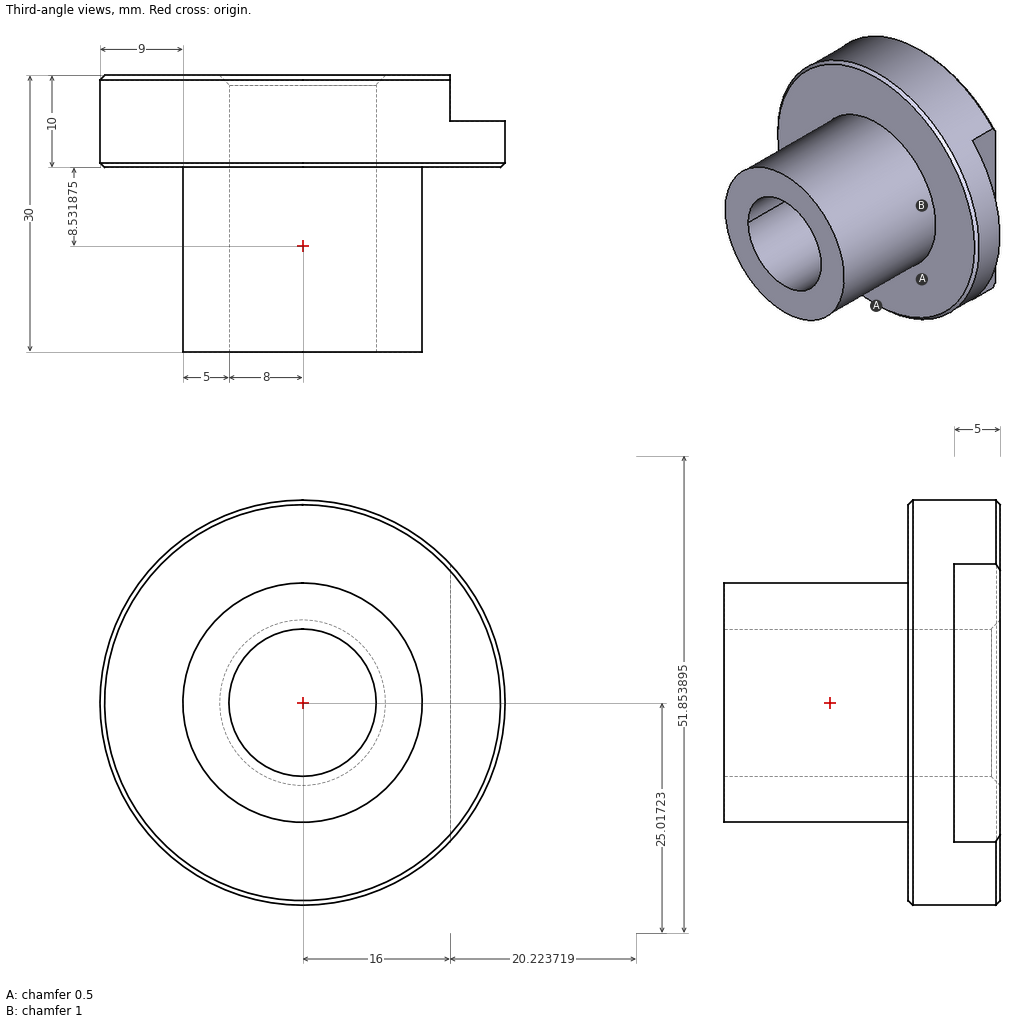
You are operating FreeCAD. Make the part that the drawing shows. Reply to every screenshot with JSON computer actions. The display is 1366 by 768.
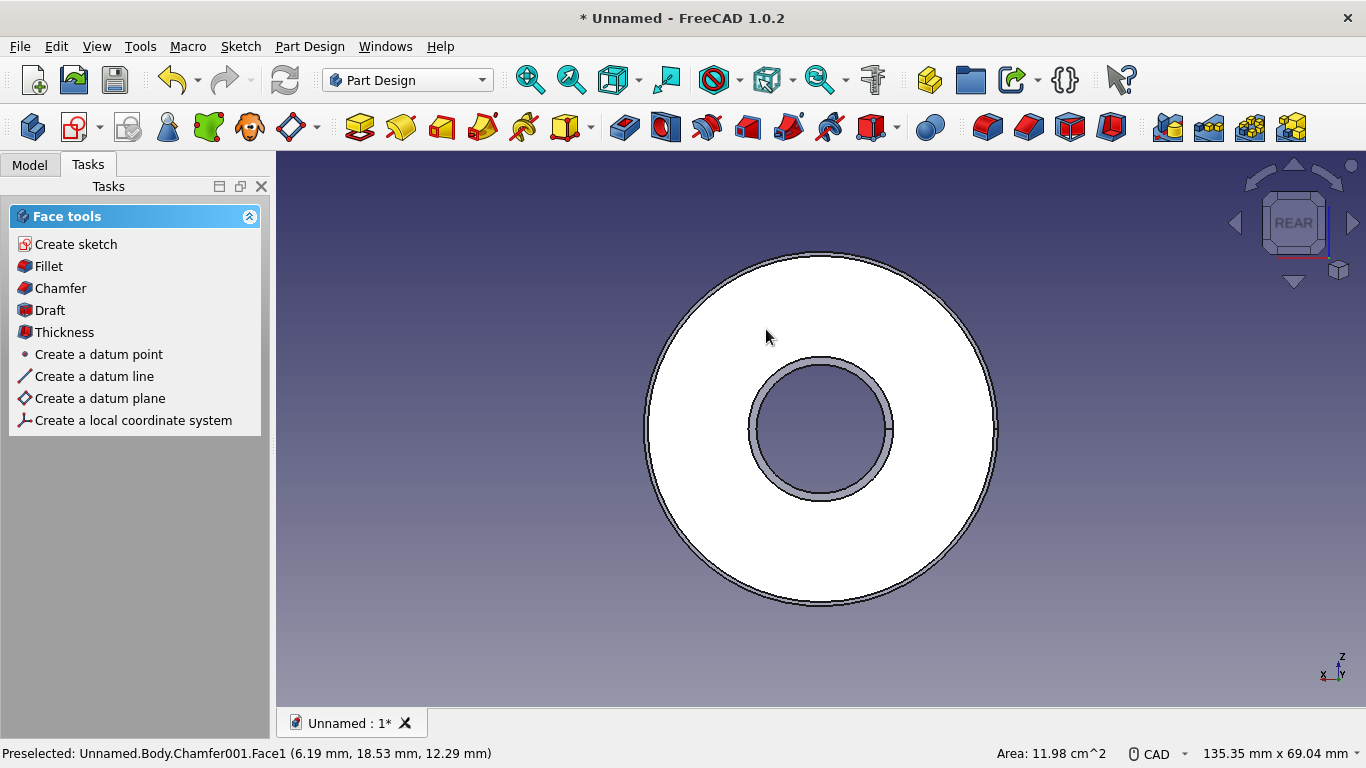
{"action": "left_click", "coordinate": [74, 128]}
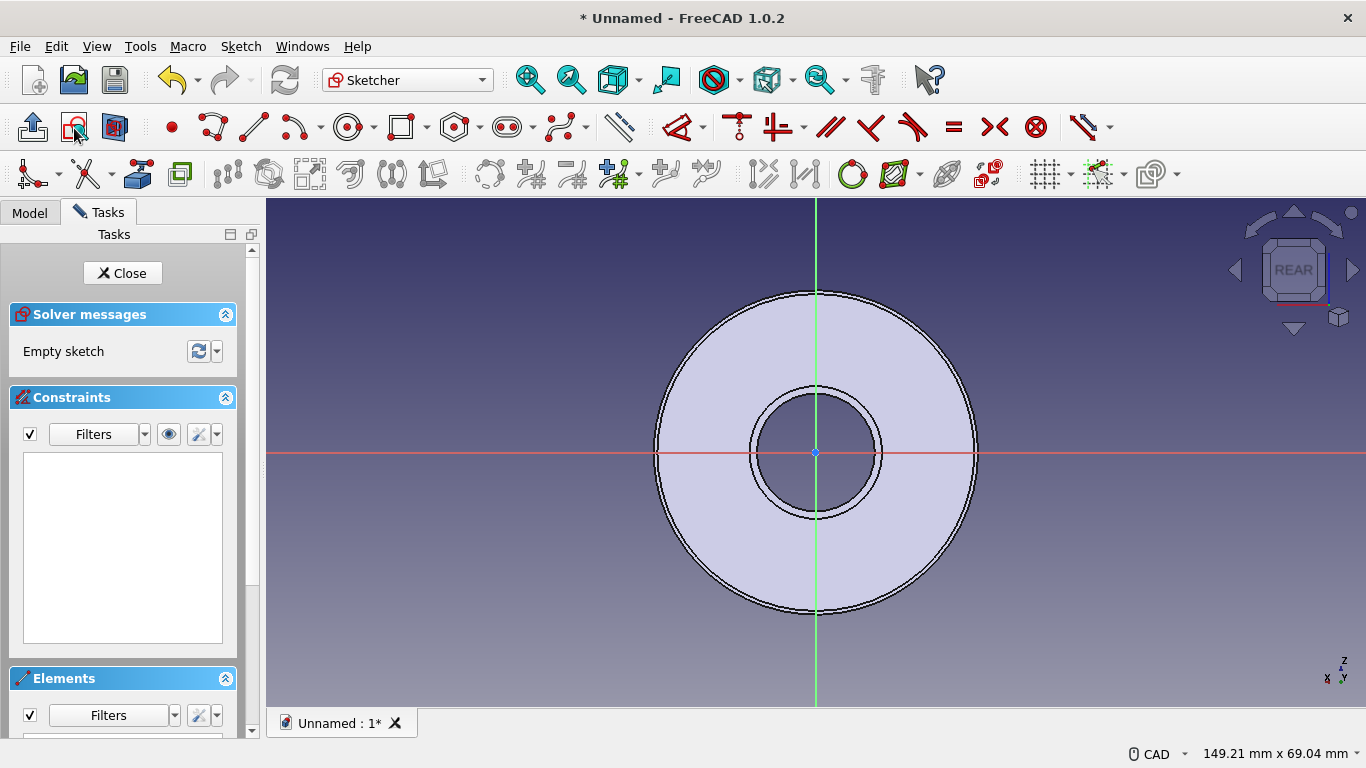
{"action": "left_click", "coordinate": [400, 128]}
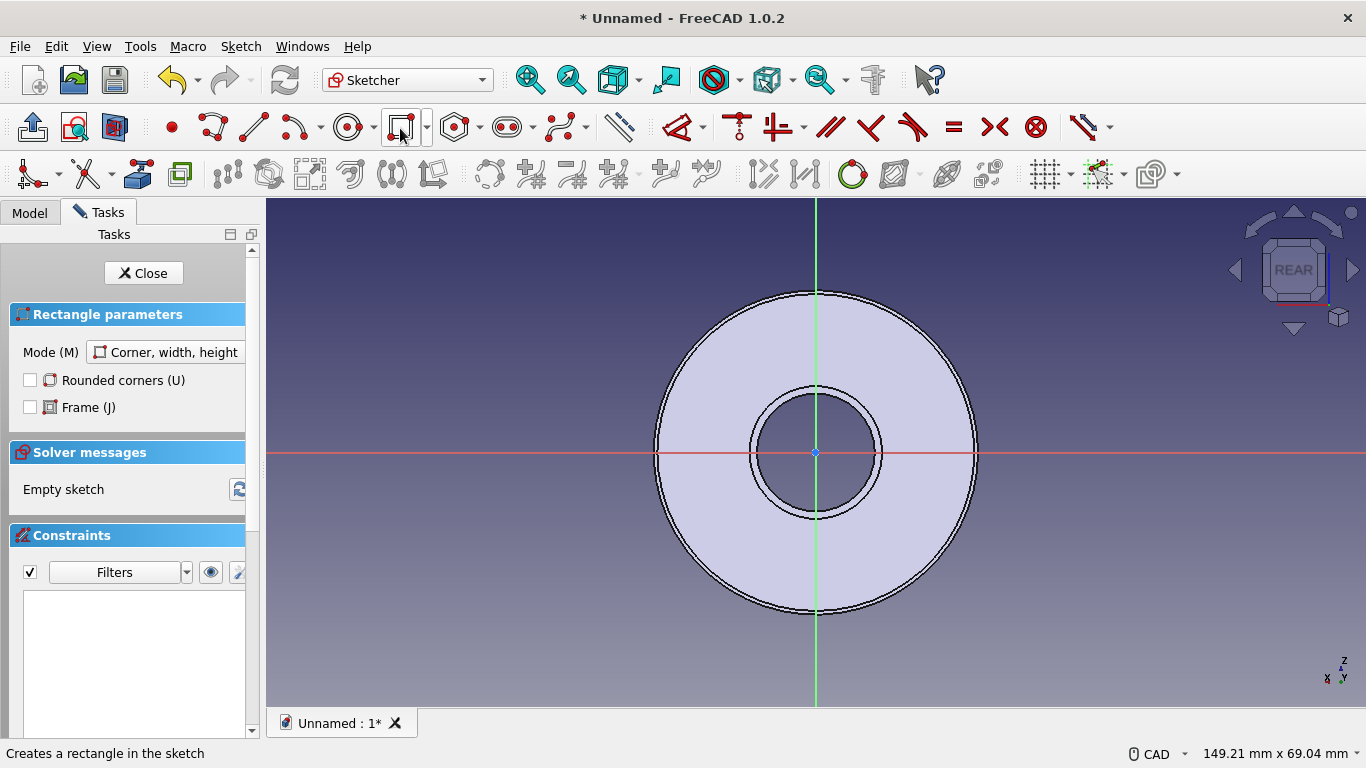
{"action": "left_click", "coordinate": [549, 255]}
{"action": "left_click", "coordinate": [698, 637]}
{"action": "key", "text": "Escape"}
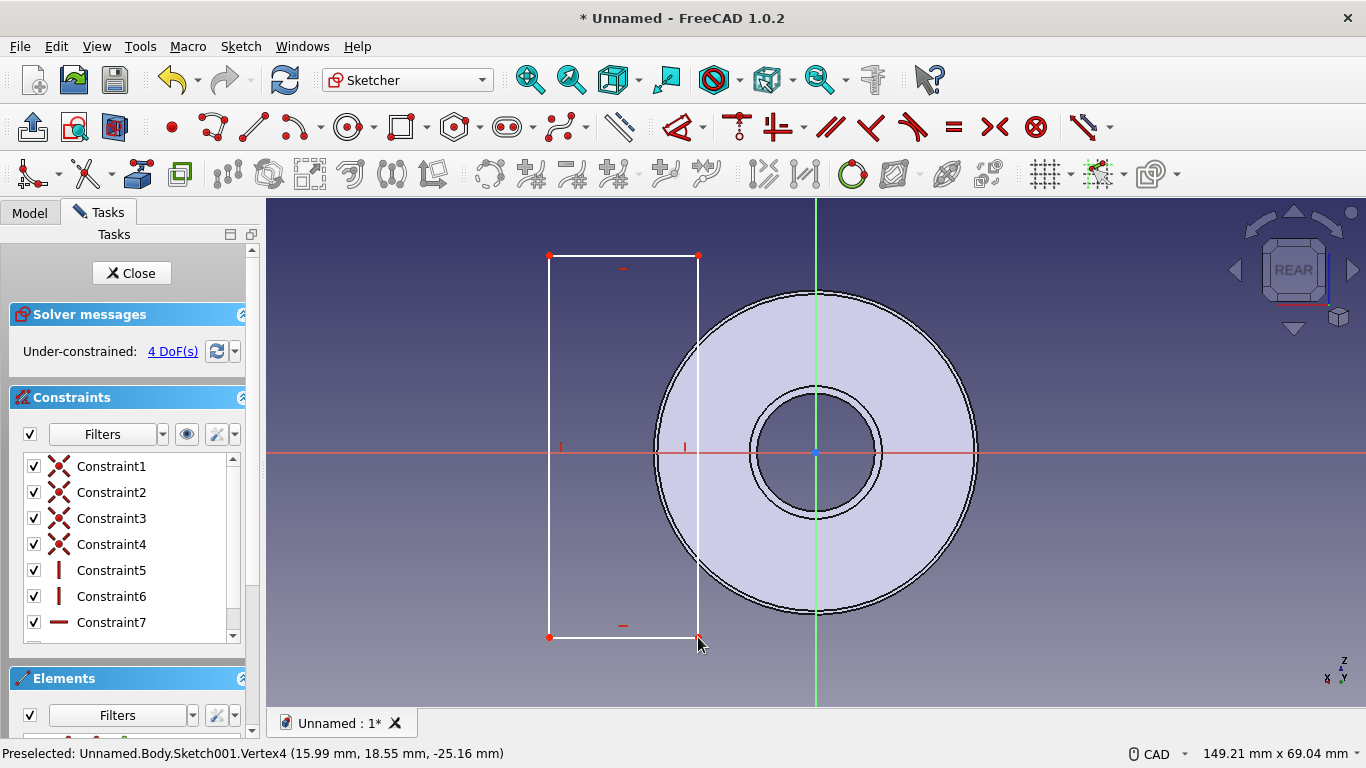
{"action": "left_click", "coordinate": [676, 128]}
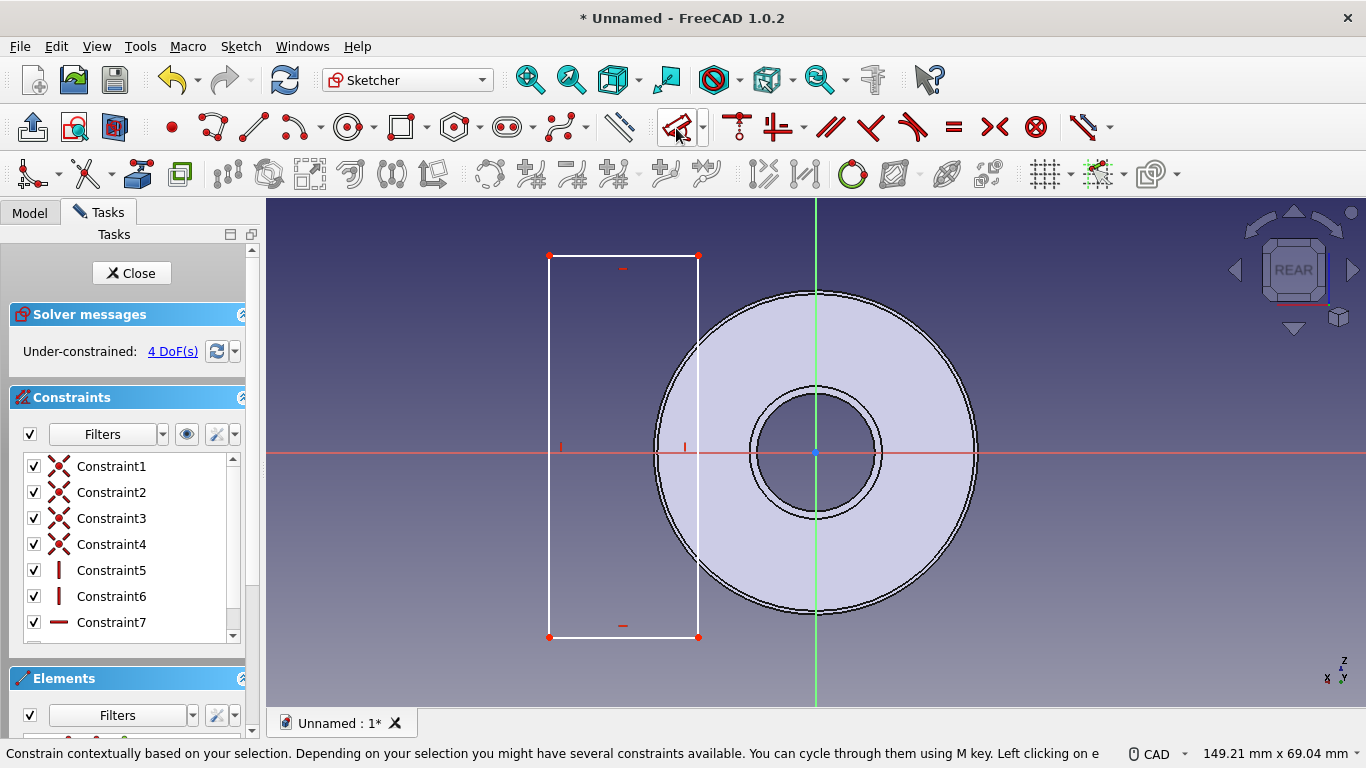
{"action": "left_click", "coordinate": [698, 638]}
{"action": "left_click", "coordinate": [757, 672]}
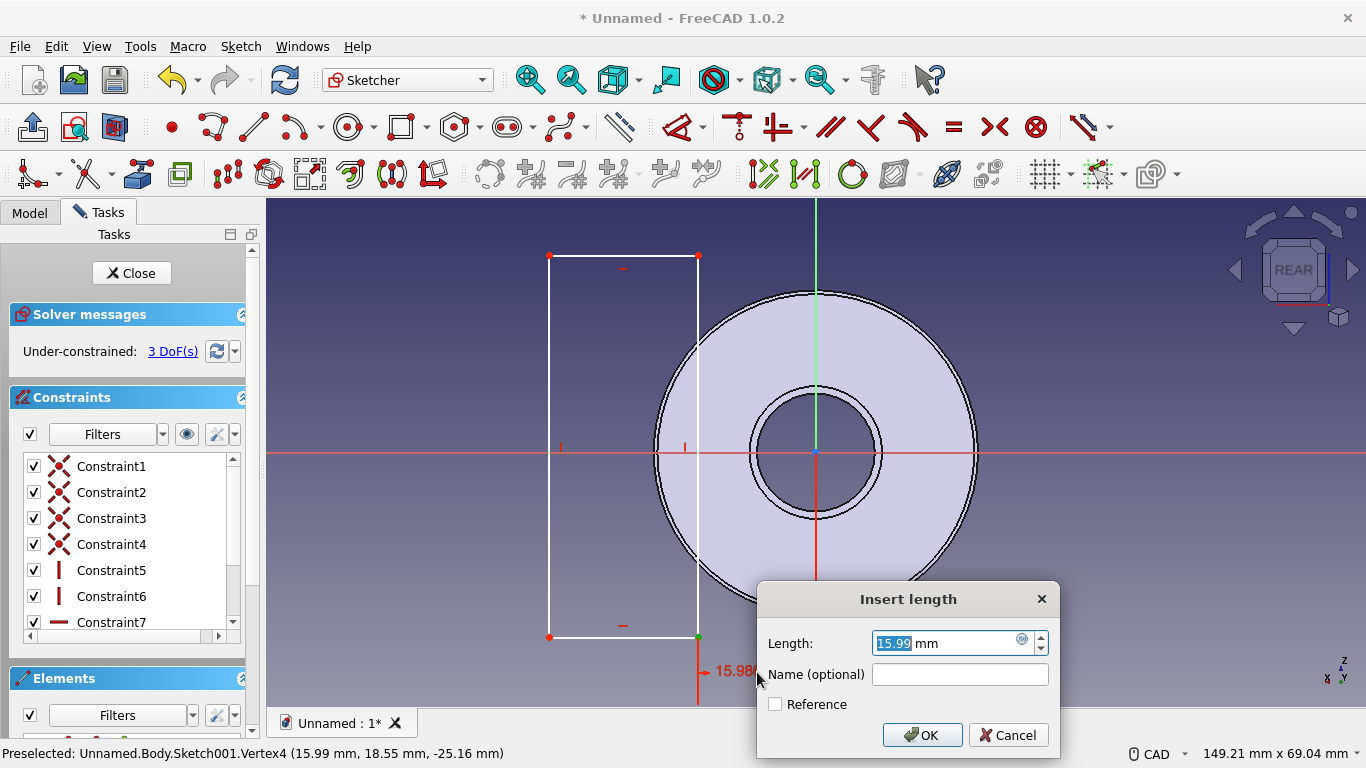
{"action": "type", "text": "16"}
{"action": "key", "text": "Return"}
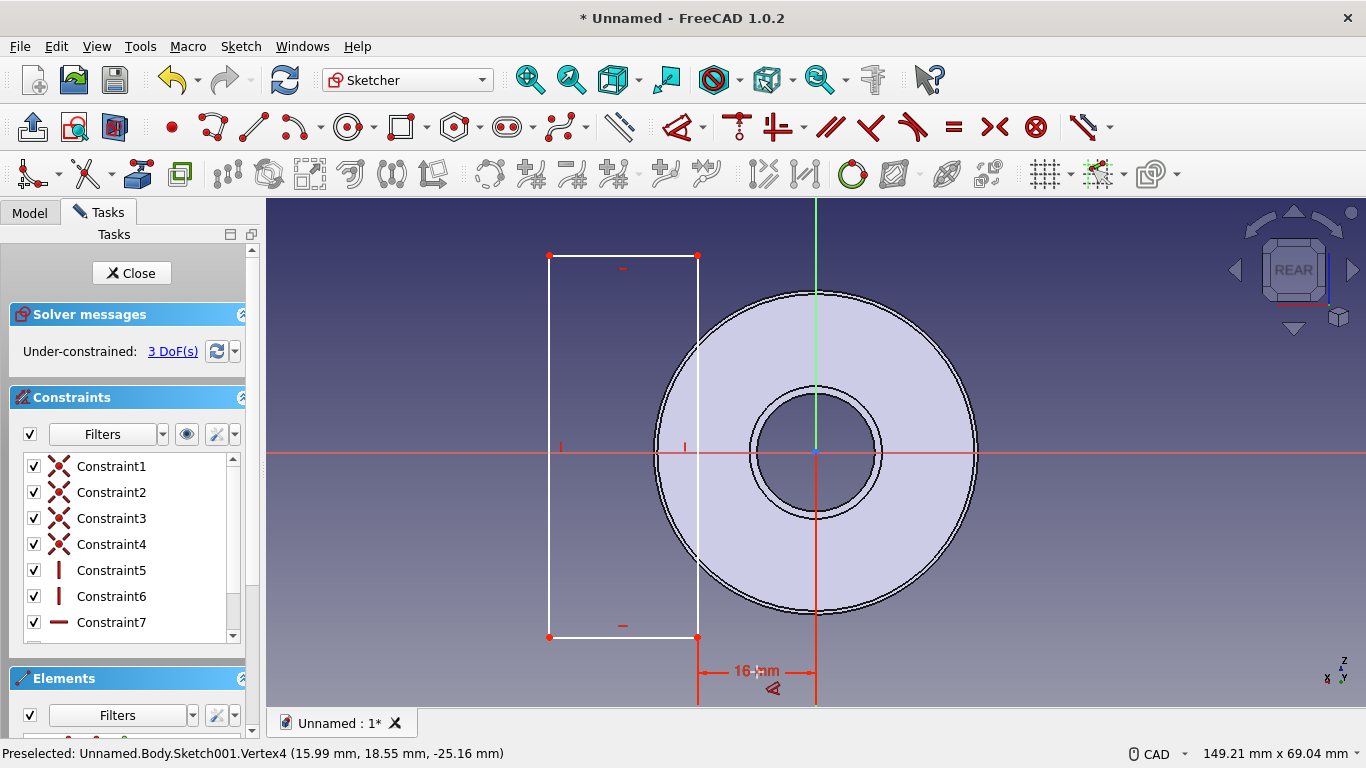
{"action": "left_click", "coordinate": [549, 371]}
{"action": "left_click", "coordinate": [515, 359]}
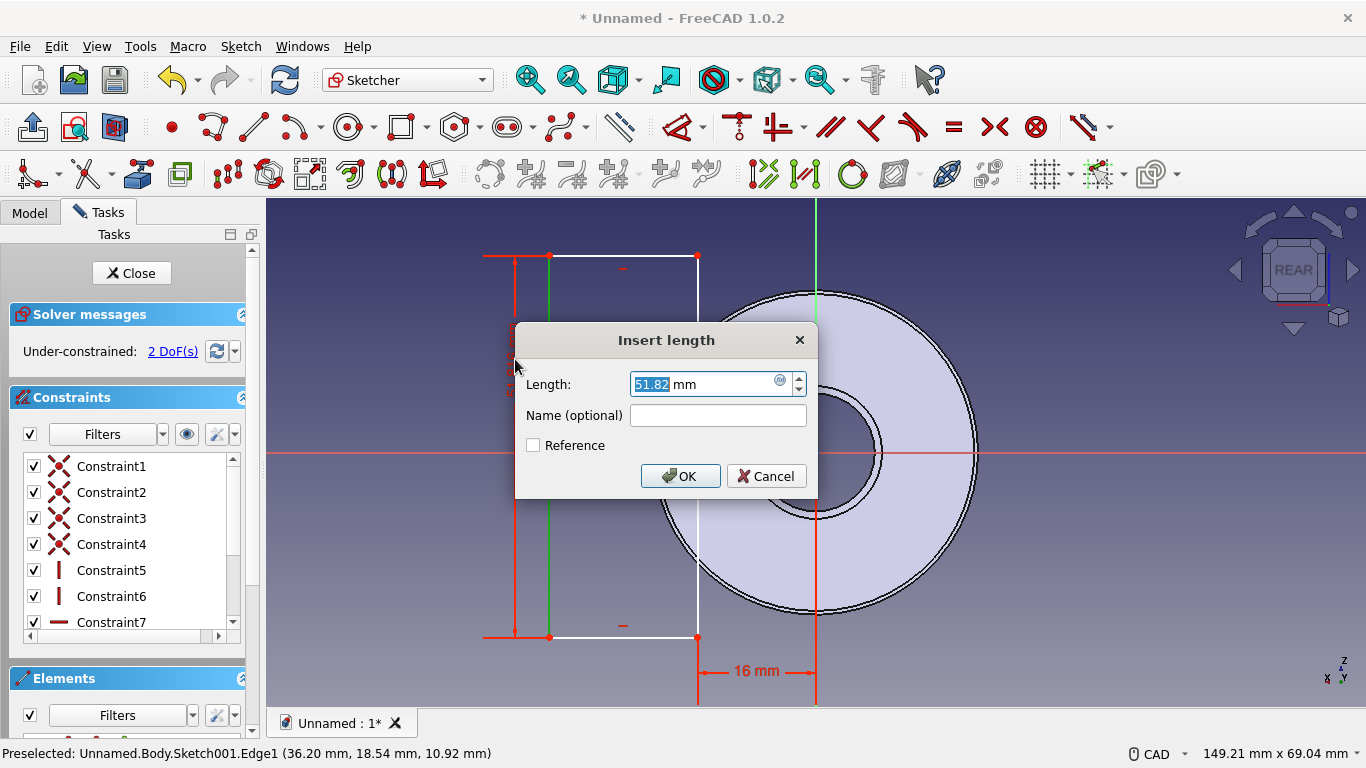
{"action": "type", "text": "51.853895"}
{"action": "key", "text": "Return"}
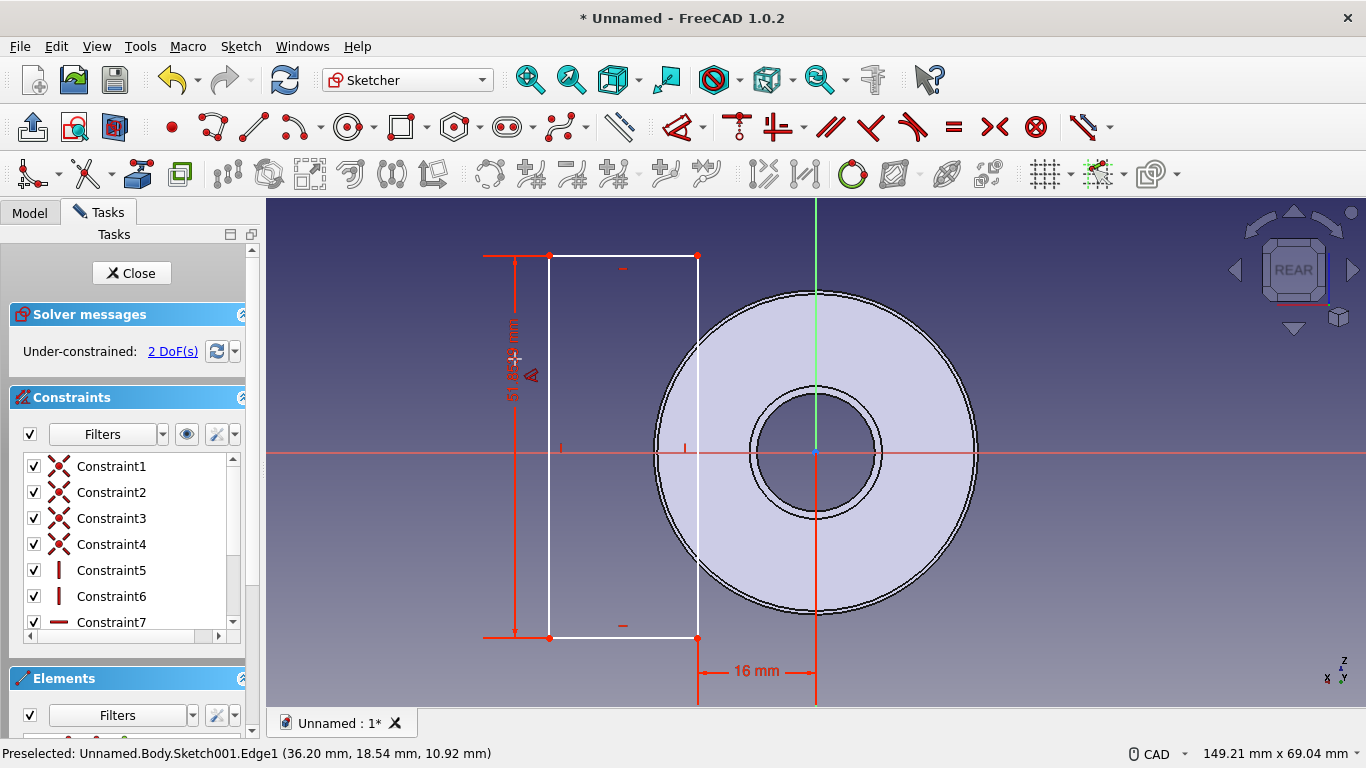
{"action": "left_click", "coordinate": [594, 638]}
{"action": "left_click", "coordinate": [623, 672]}